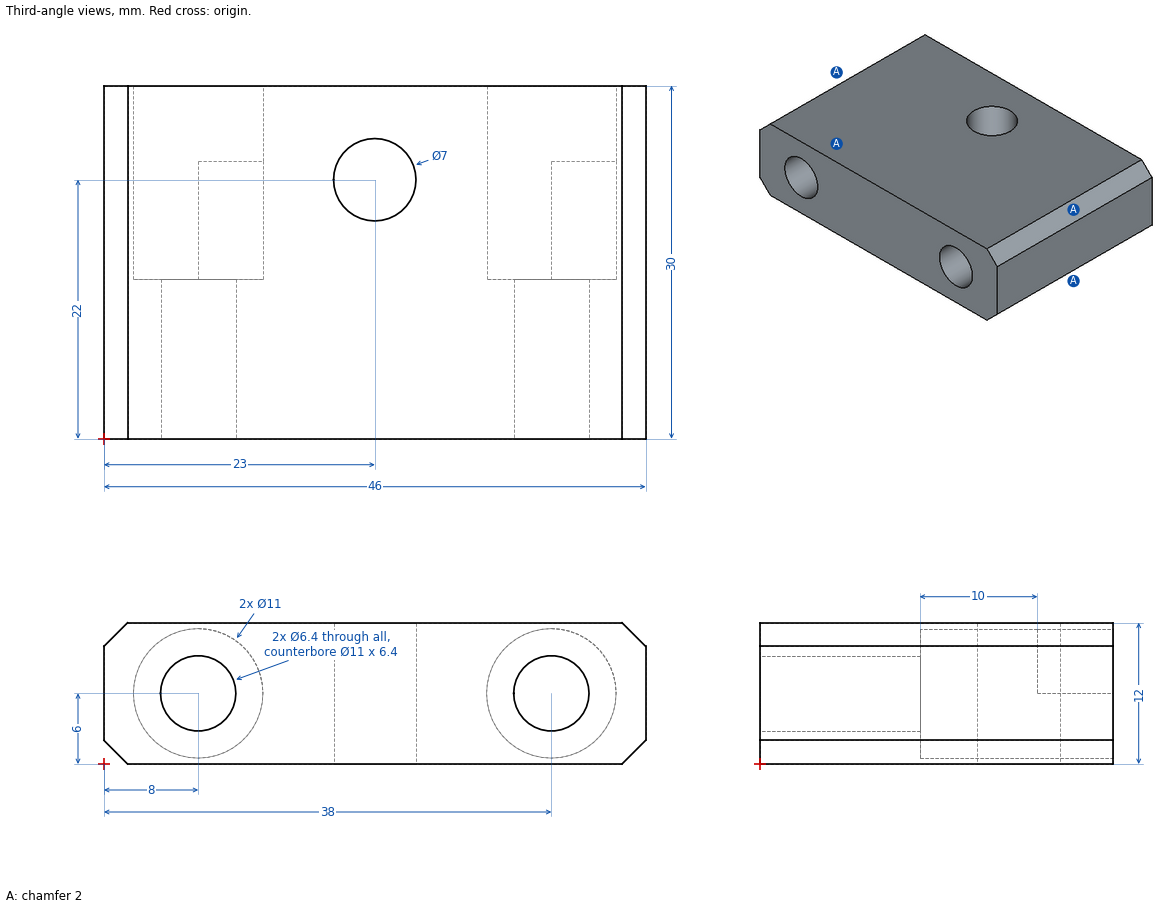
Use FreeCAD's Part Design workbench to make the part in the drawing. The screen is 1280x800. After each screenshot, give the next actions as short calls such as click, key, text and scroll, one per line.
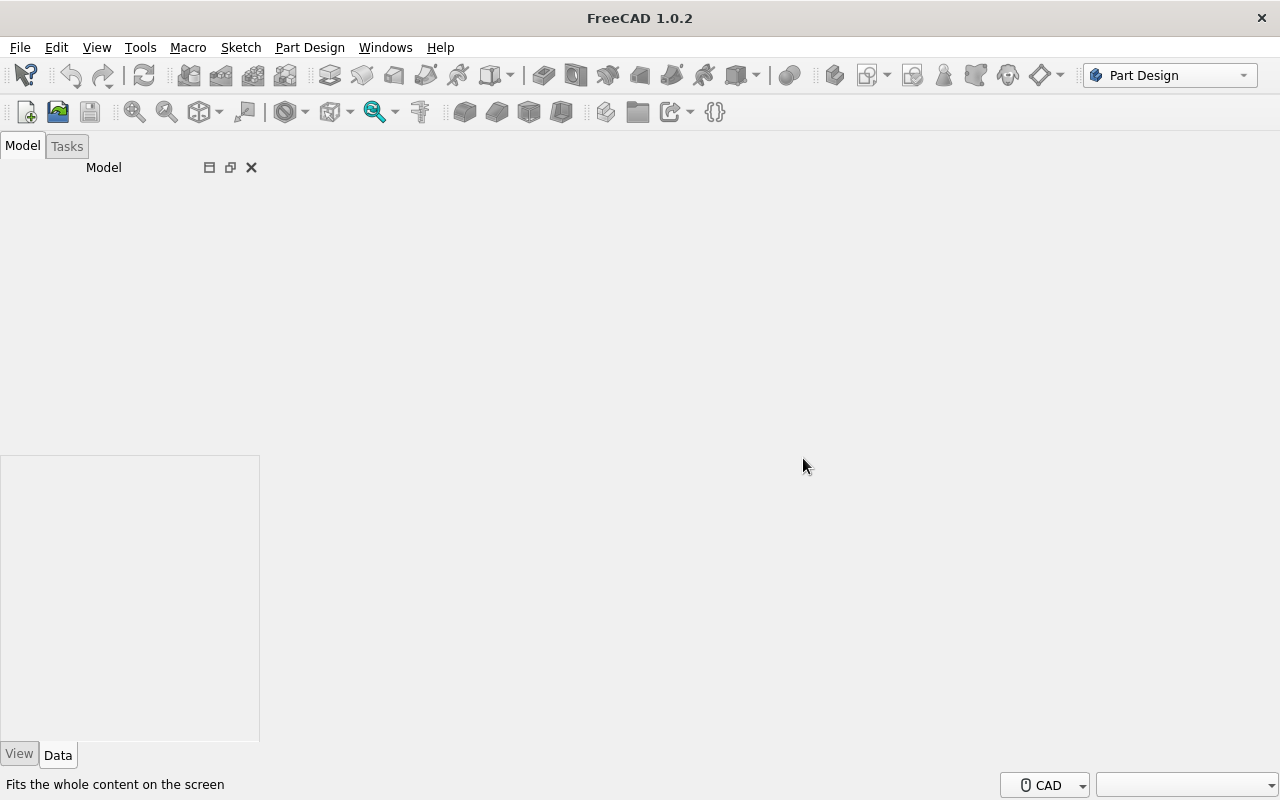
click(26, 112)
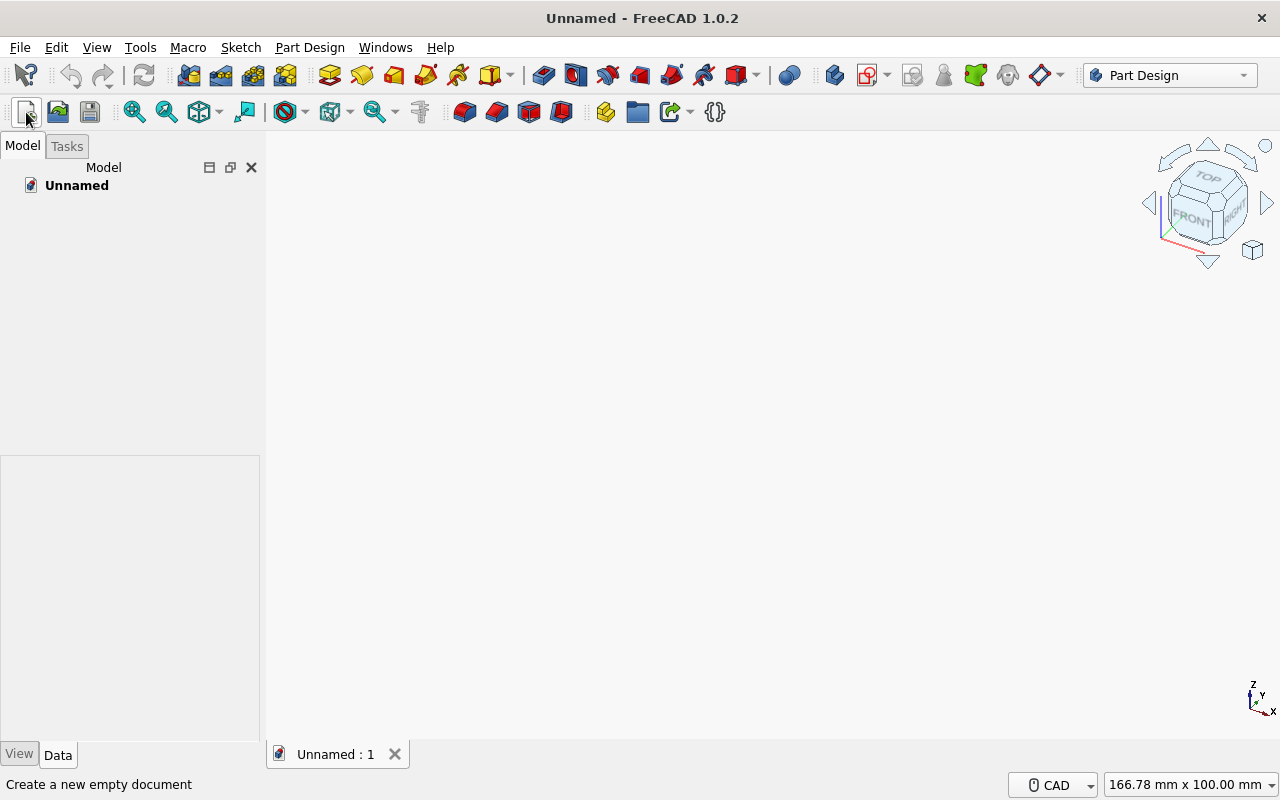
click(868, 76)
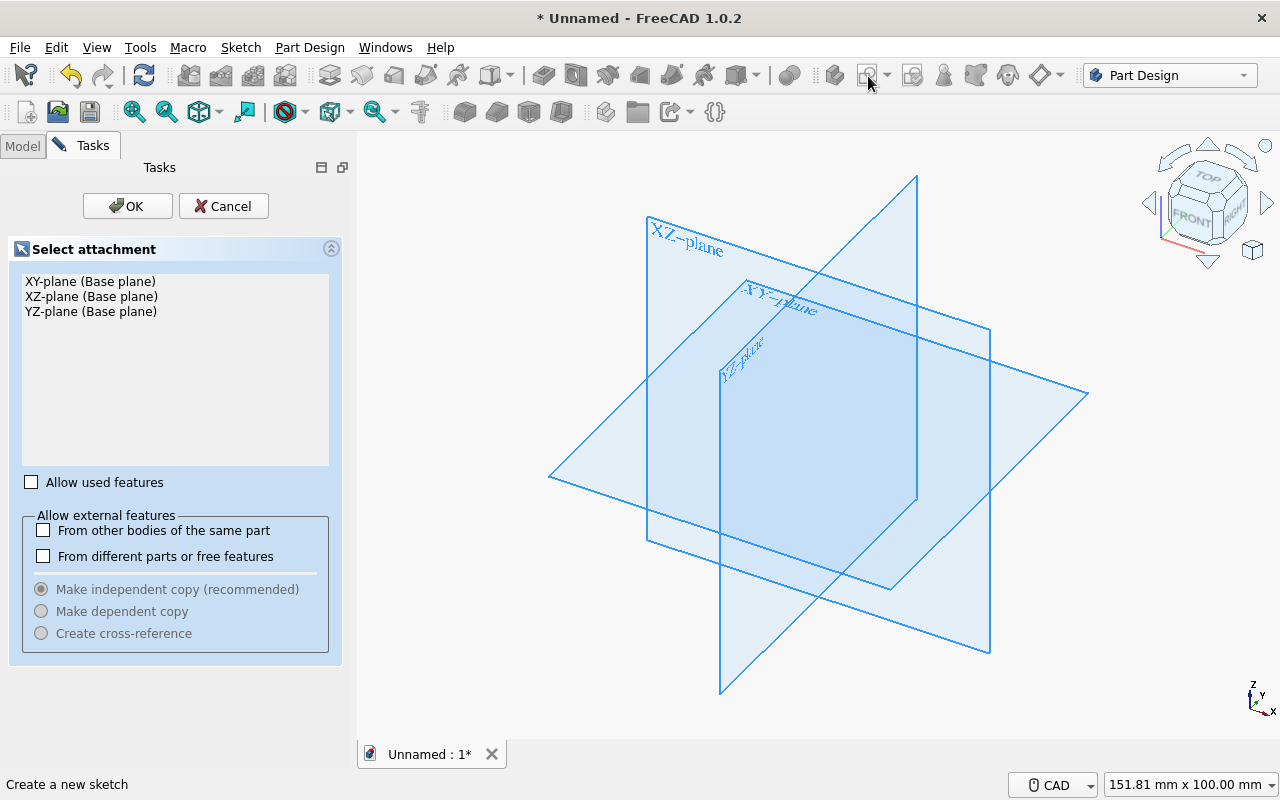
click(82, 282)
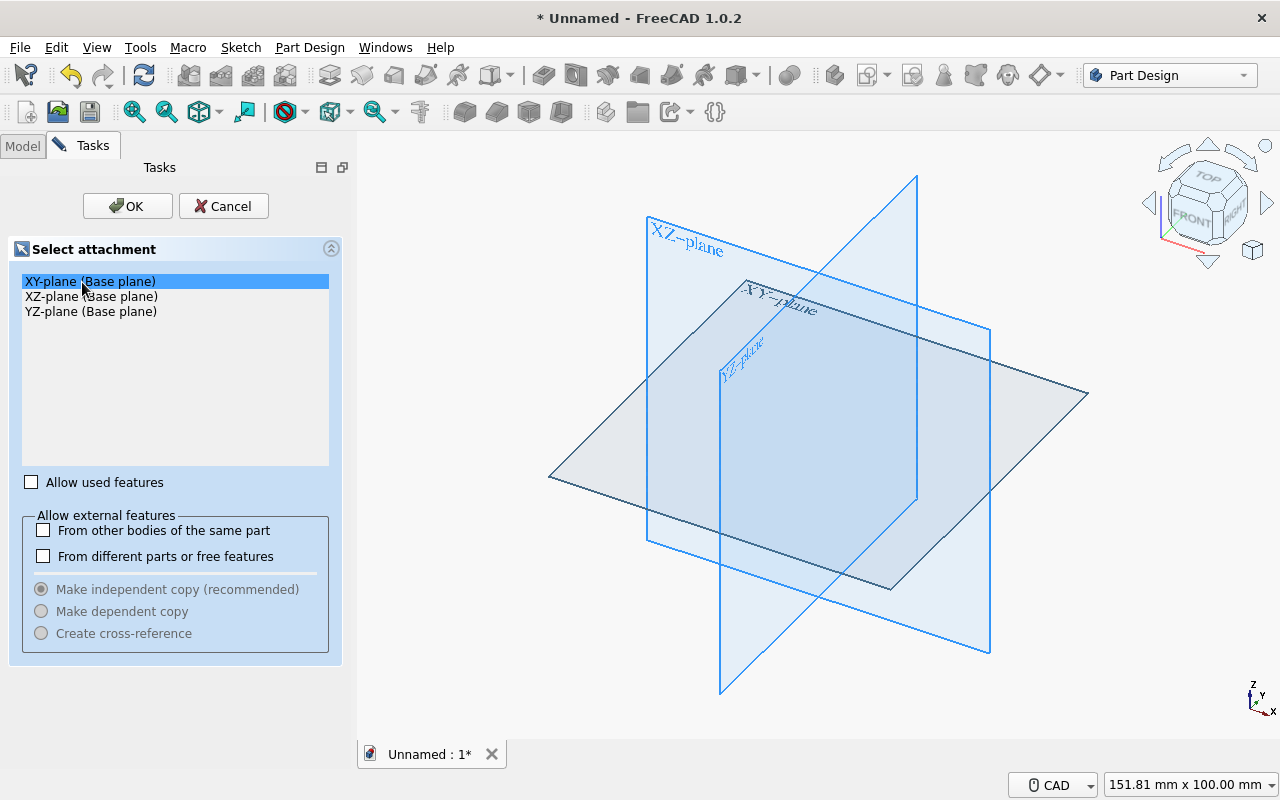
click(128, 206)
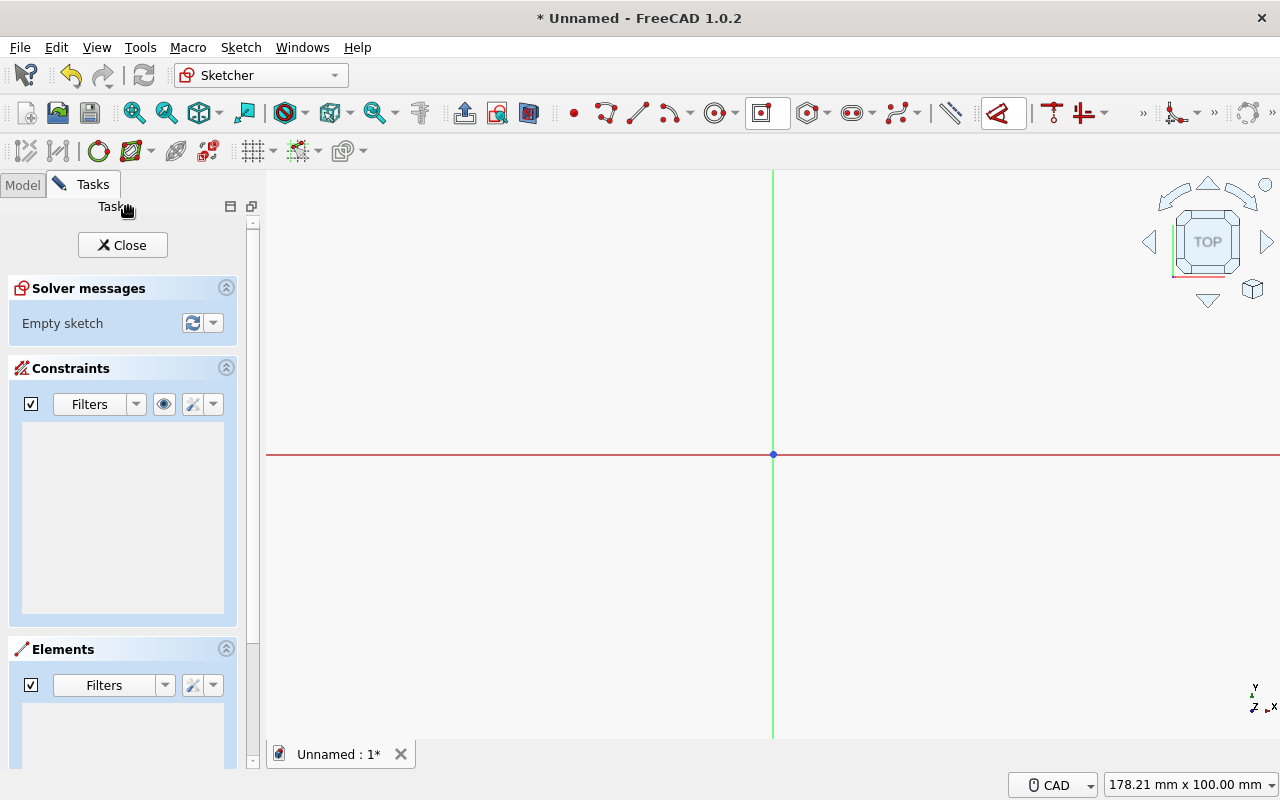
scroll(1067, 300, up, 4)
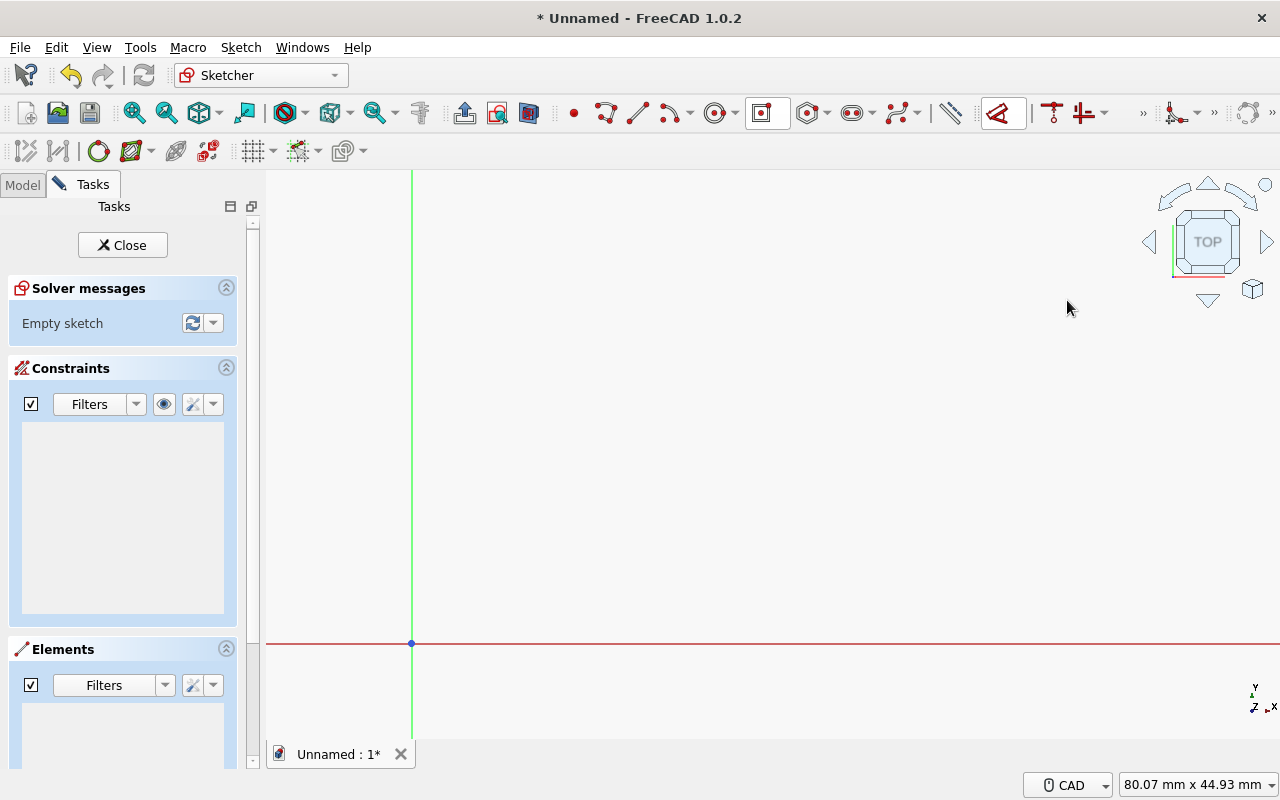
key(g)
key(r)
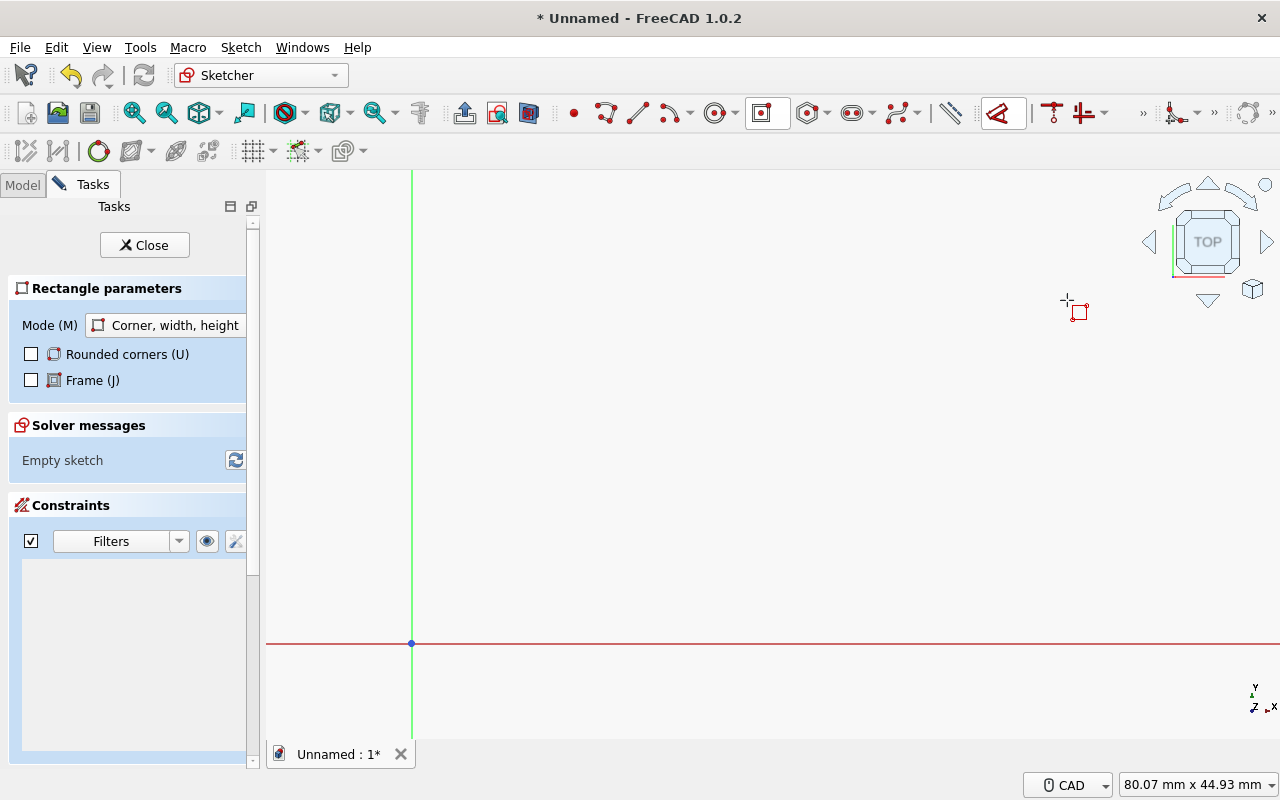
click(412, 644)
move(994, 264)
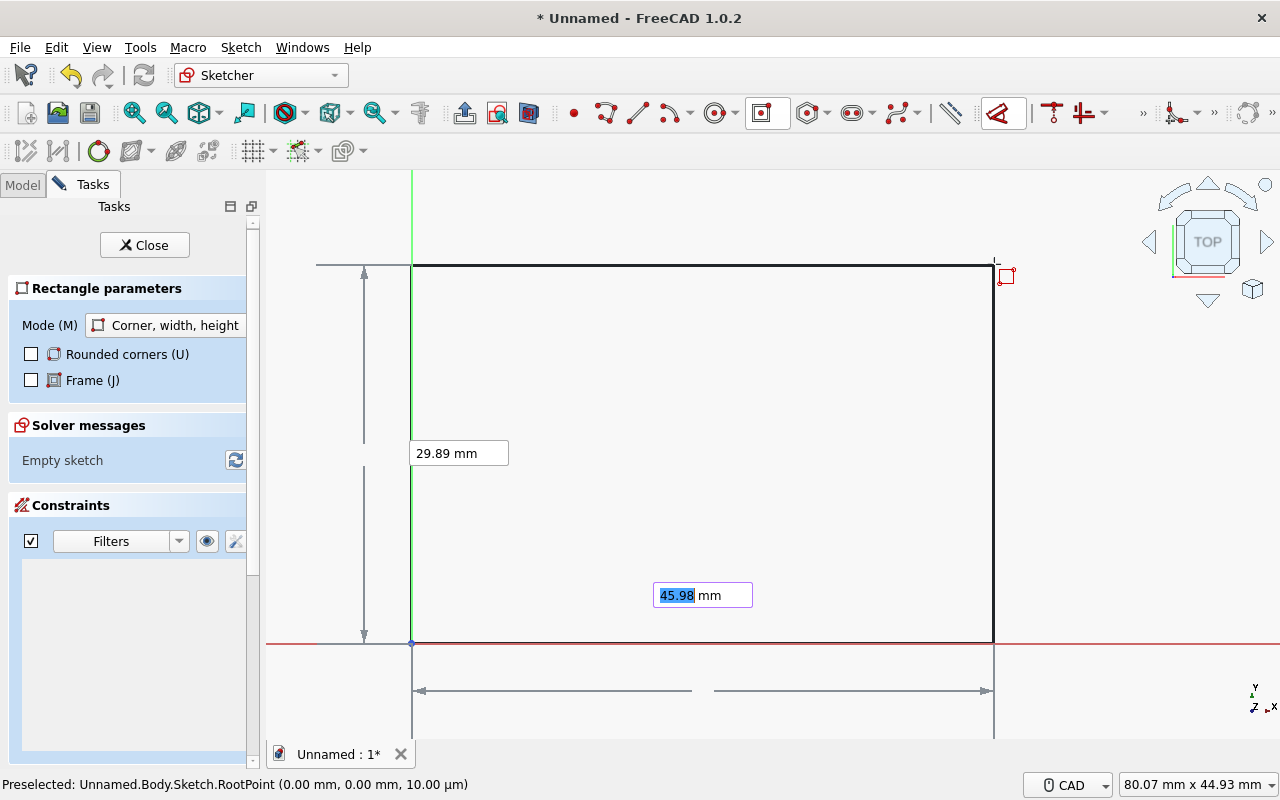
text(46)
key(Tab)
text(30)
key(Return)
key(Escape)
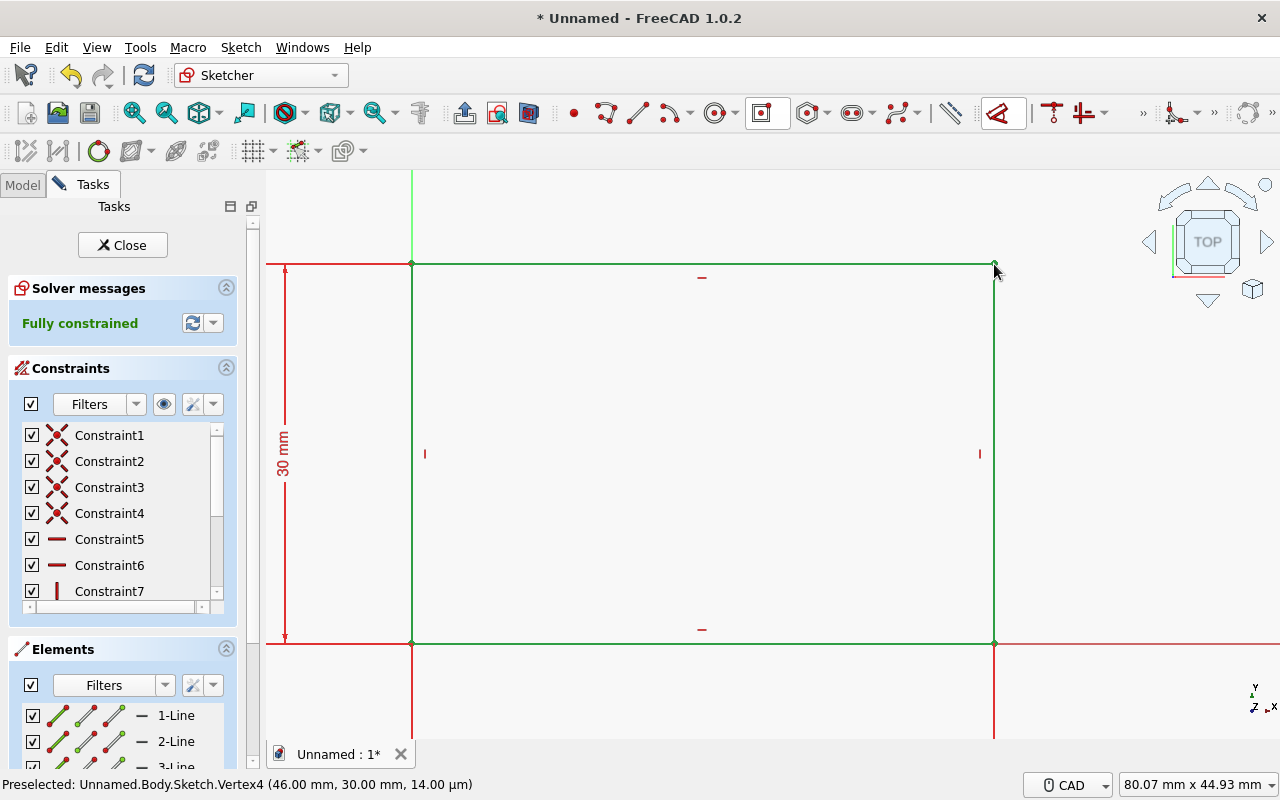
click(123, 245)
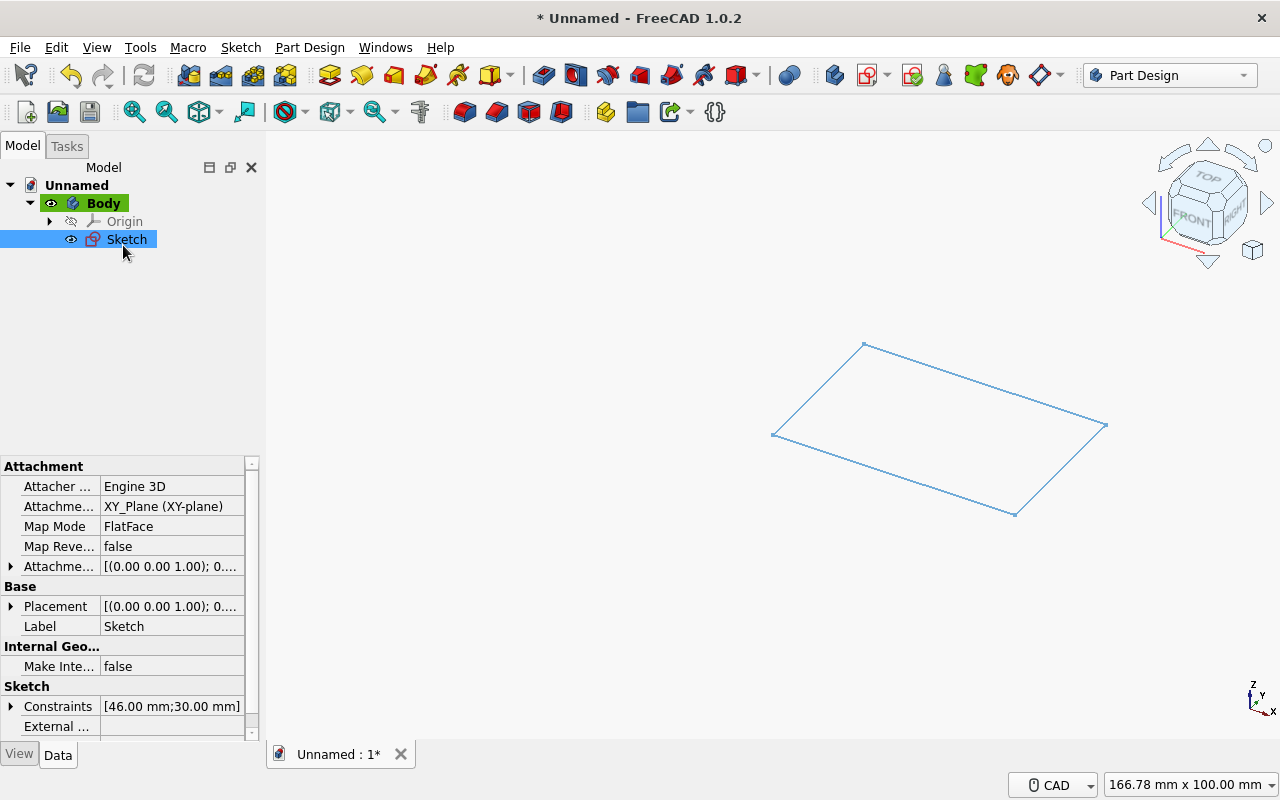
click(330, 76)